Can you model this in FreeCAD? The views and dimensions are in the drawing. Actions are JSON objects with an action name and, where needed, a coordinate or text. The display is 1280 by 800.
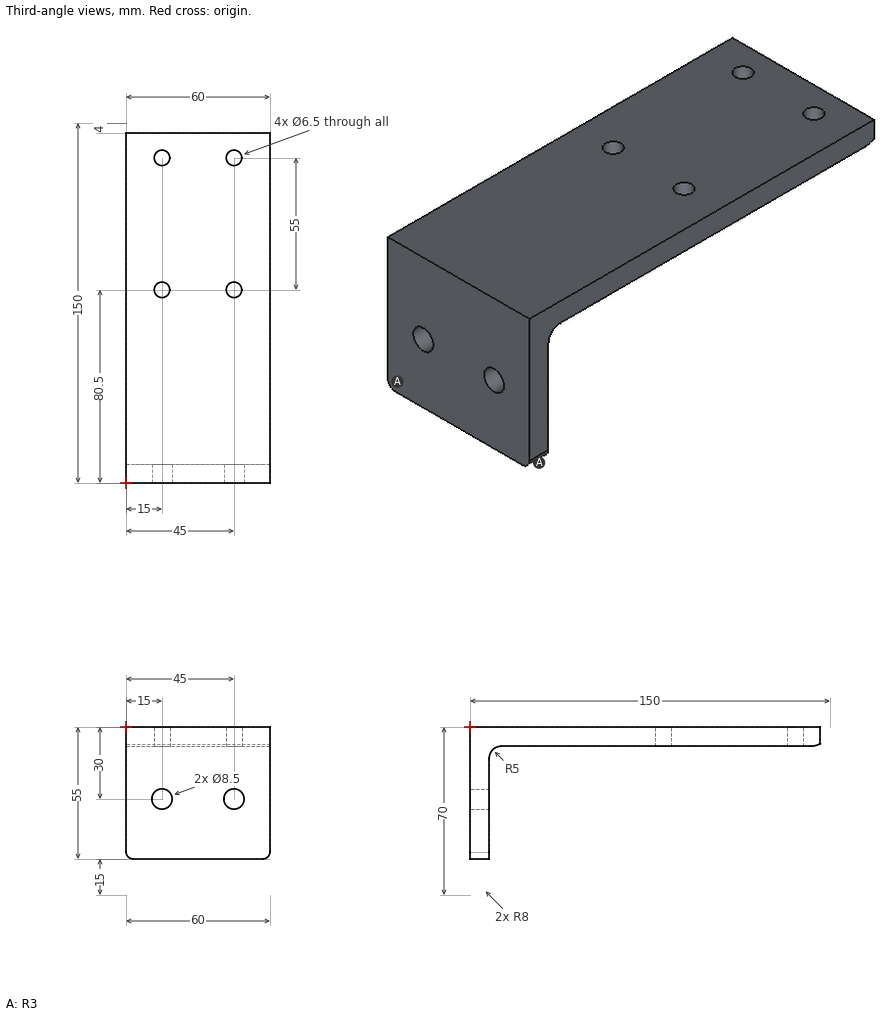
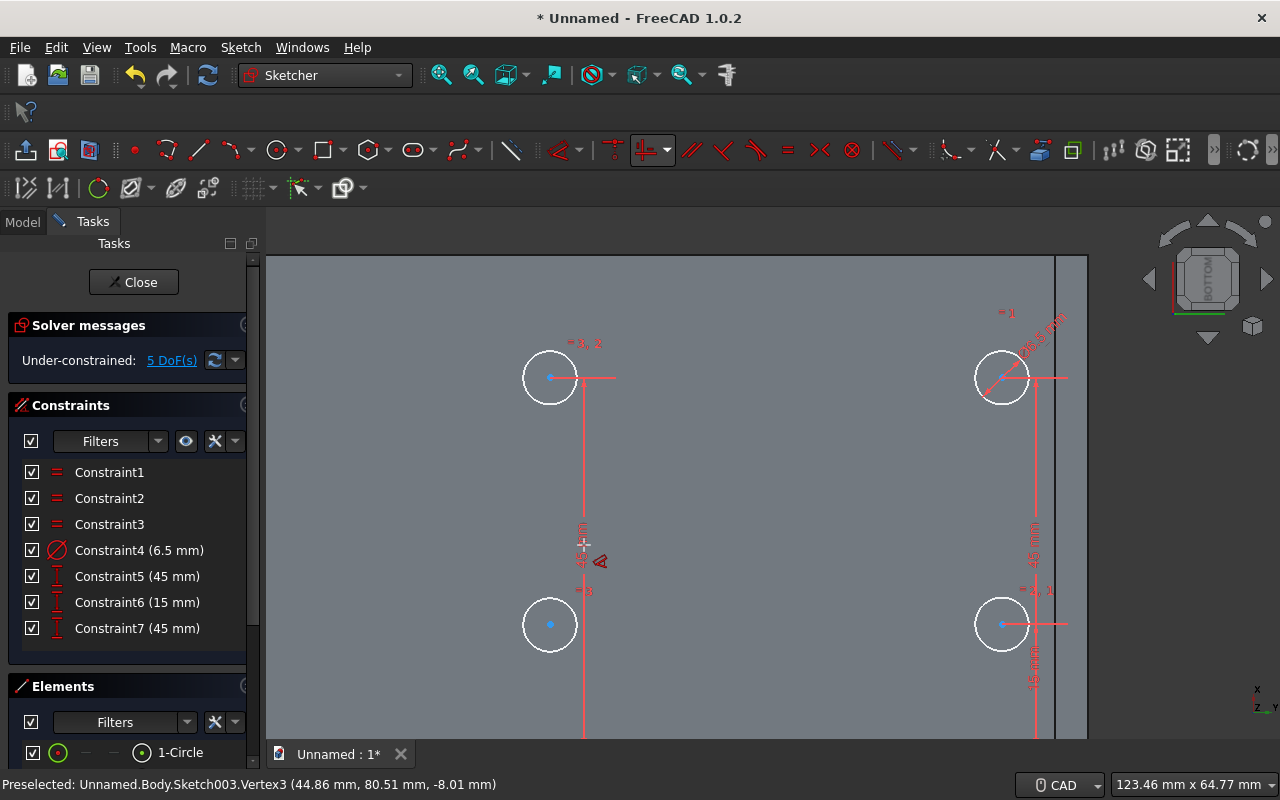
{"action": "left_click", "coordinate": [550, 625]}
{"action": "left_click", "coordinate": [584, 668]}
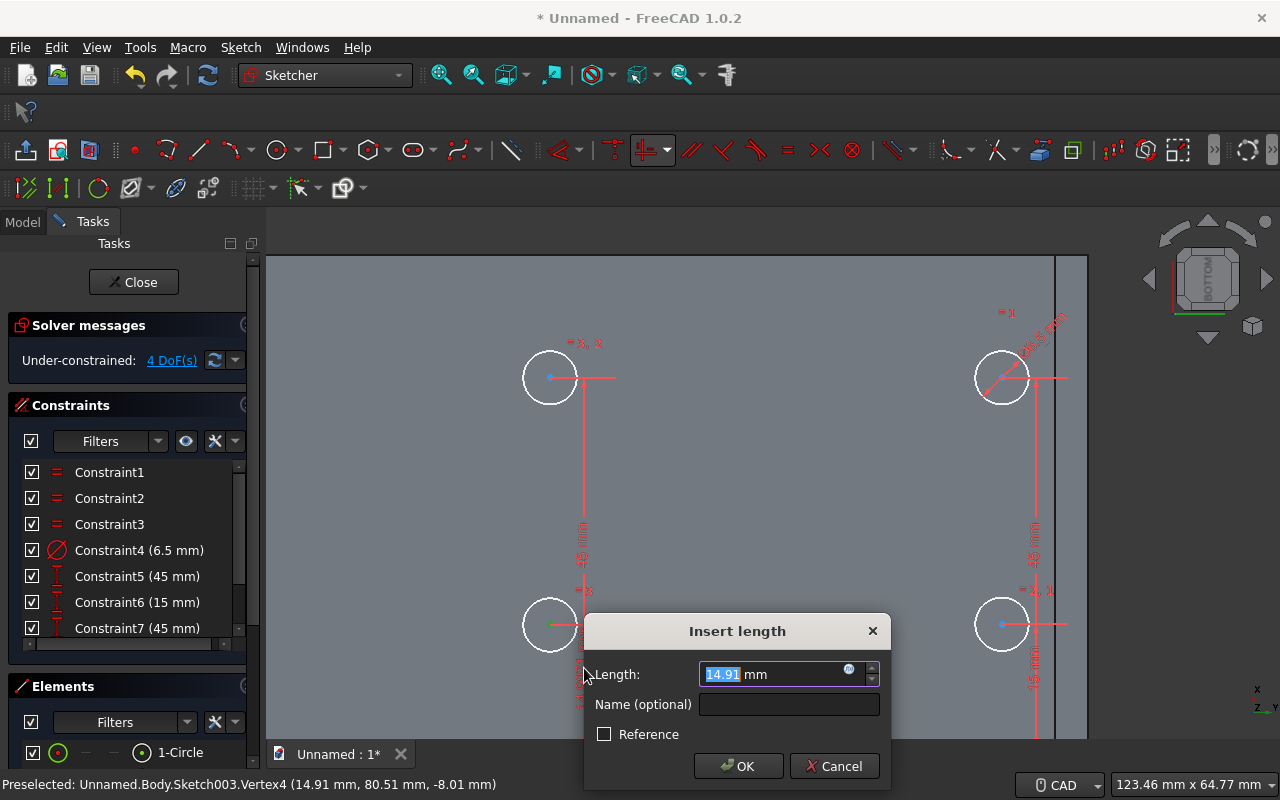
{"action": "type", "text": "15"}
{"action": "key", "text": "Return"}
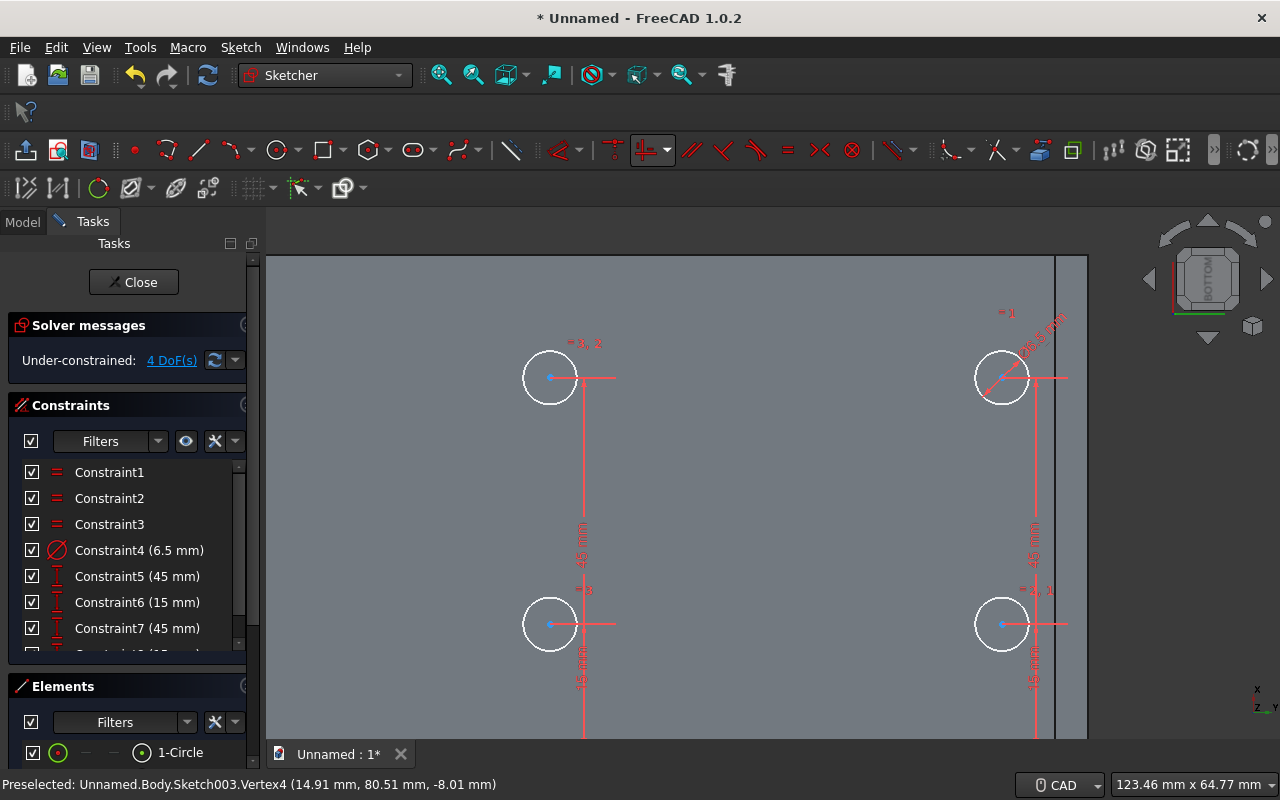
{"action": "left_click", "coordinate": [1002, 378]}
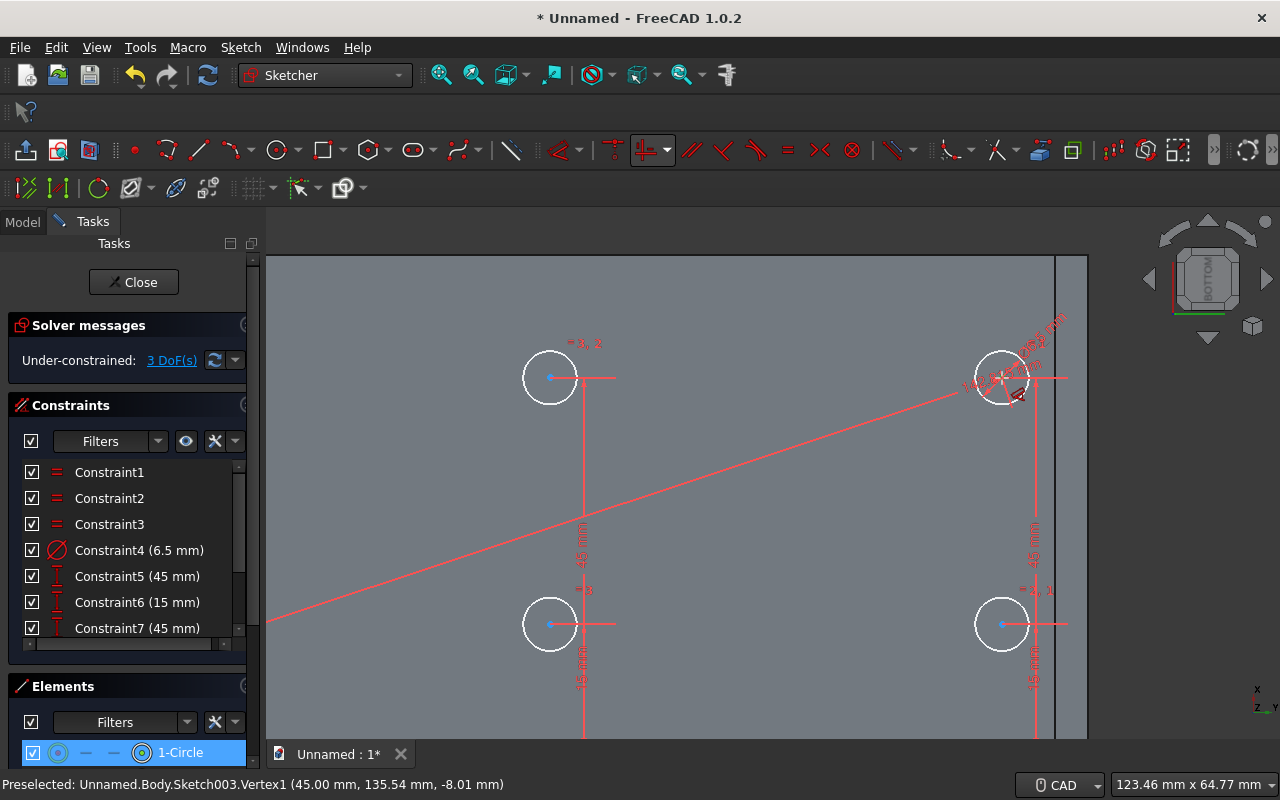
{"action": "left_click", "coordinate": [550, 378]}
{"action": "left_click", "coordinate": [776, 344]}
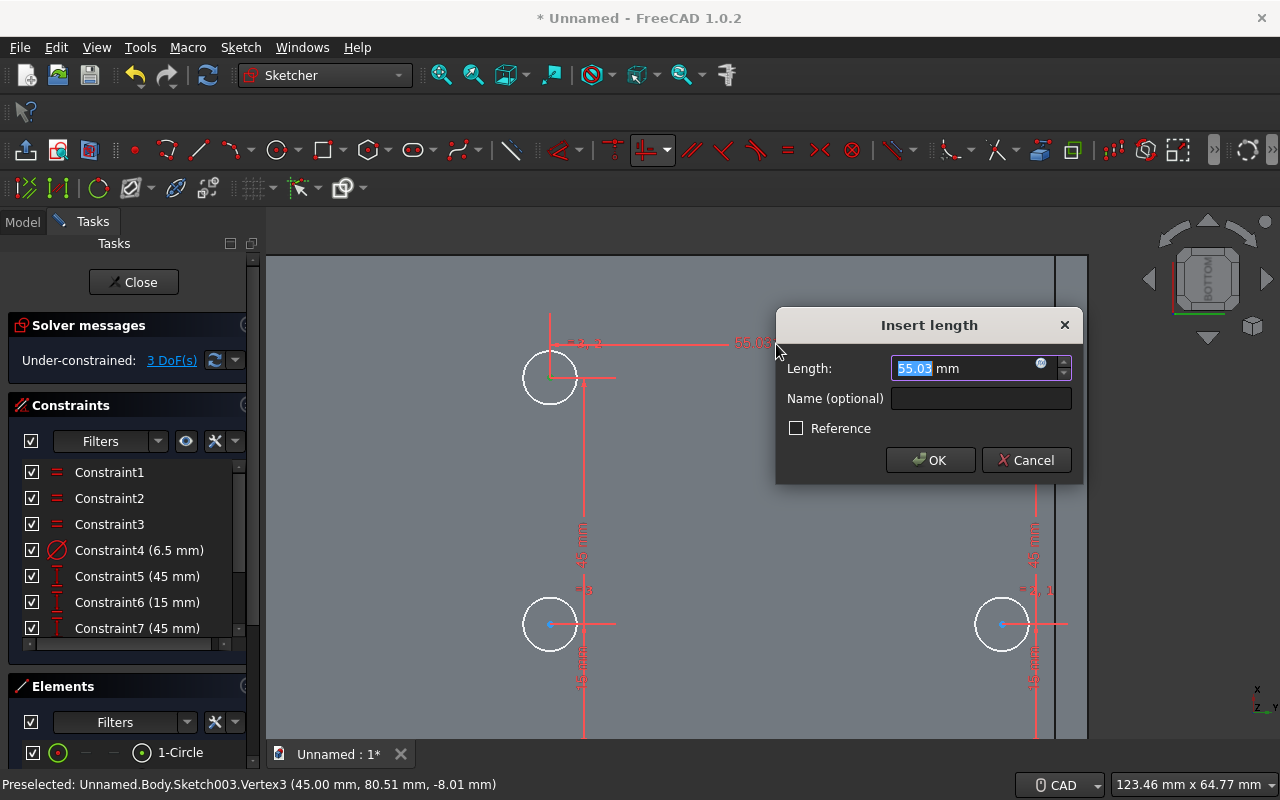
{"action": "type", "text": "55"}
{"action": "key", "text": "Return"}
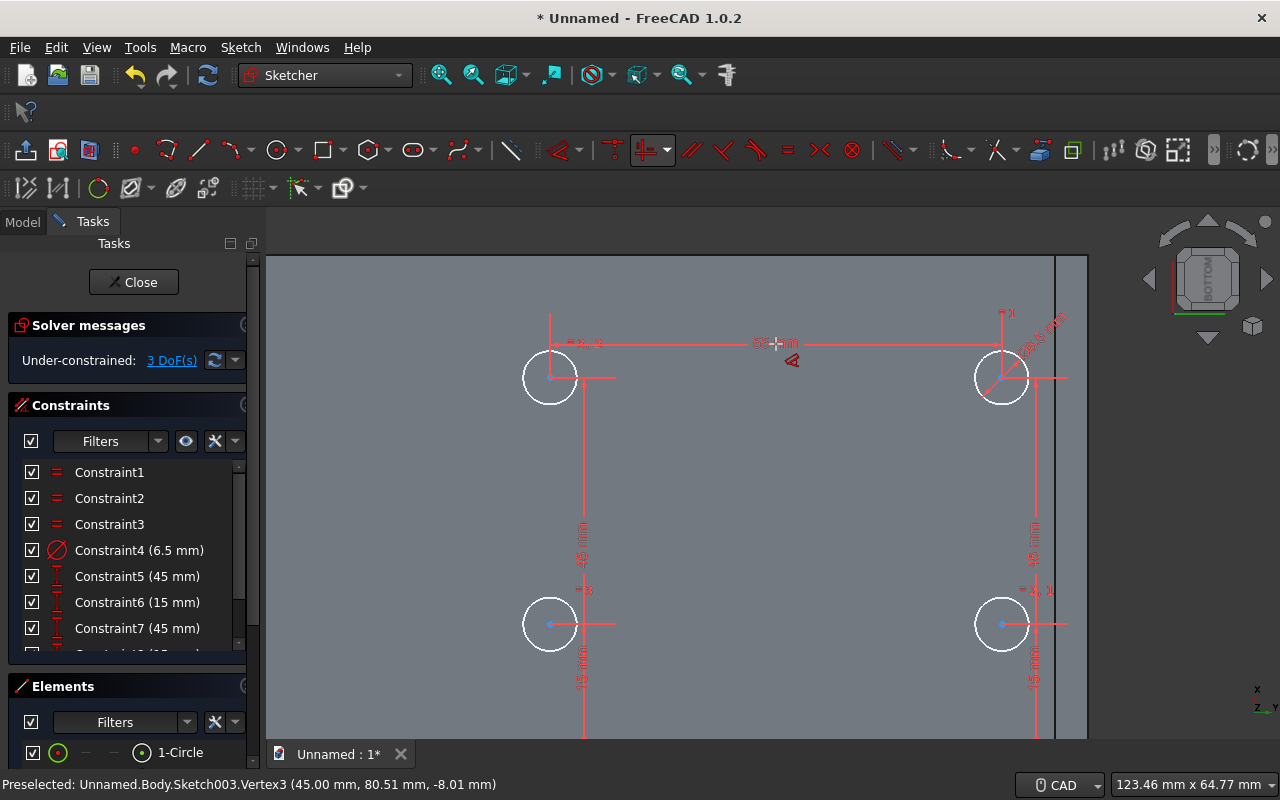
{"action": "left_click", "coordinate": [1002, 624]}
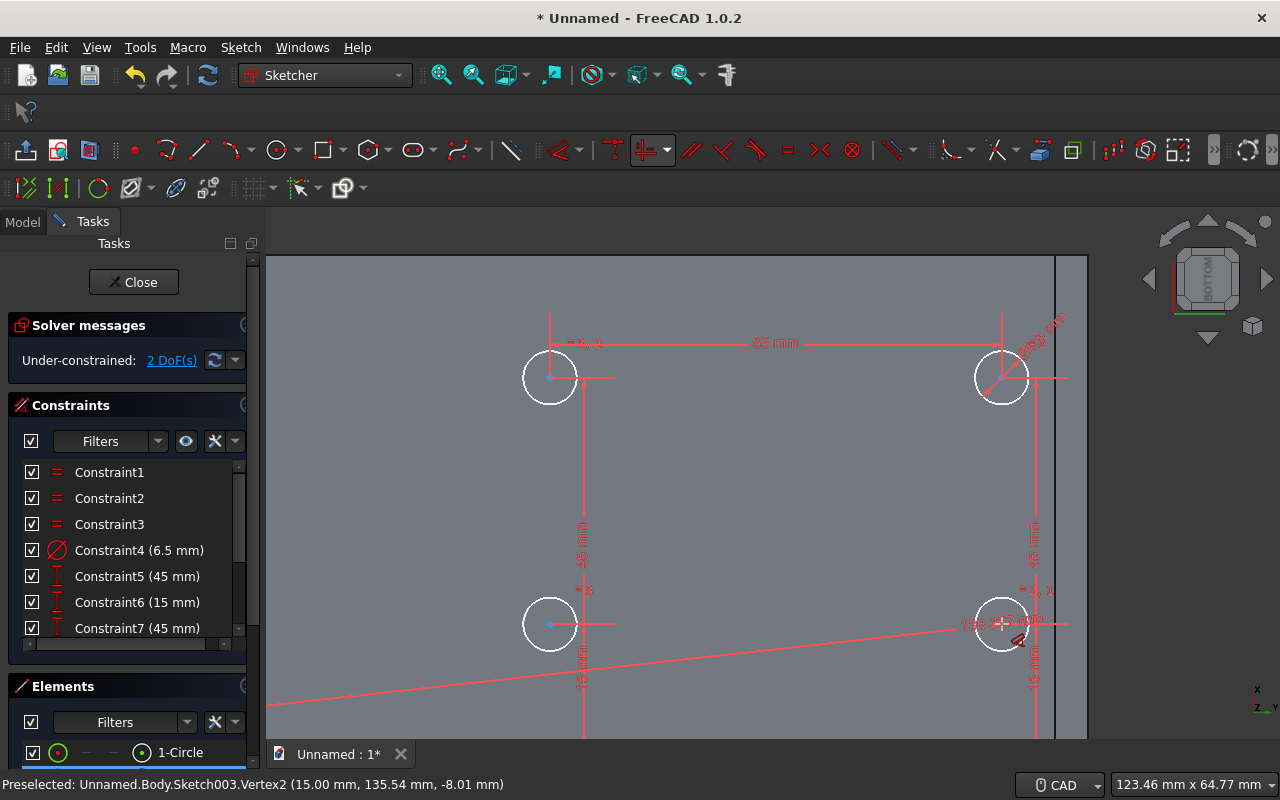
{"action": "left_click", "coordinate": [550, 378]}
{"action": "left_click", "coordinate": [672, 344]}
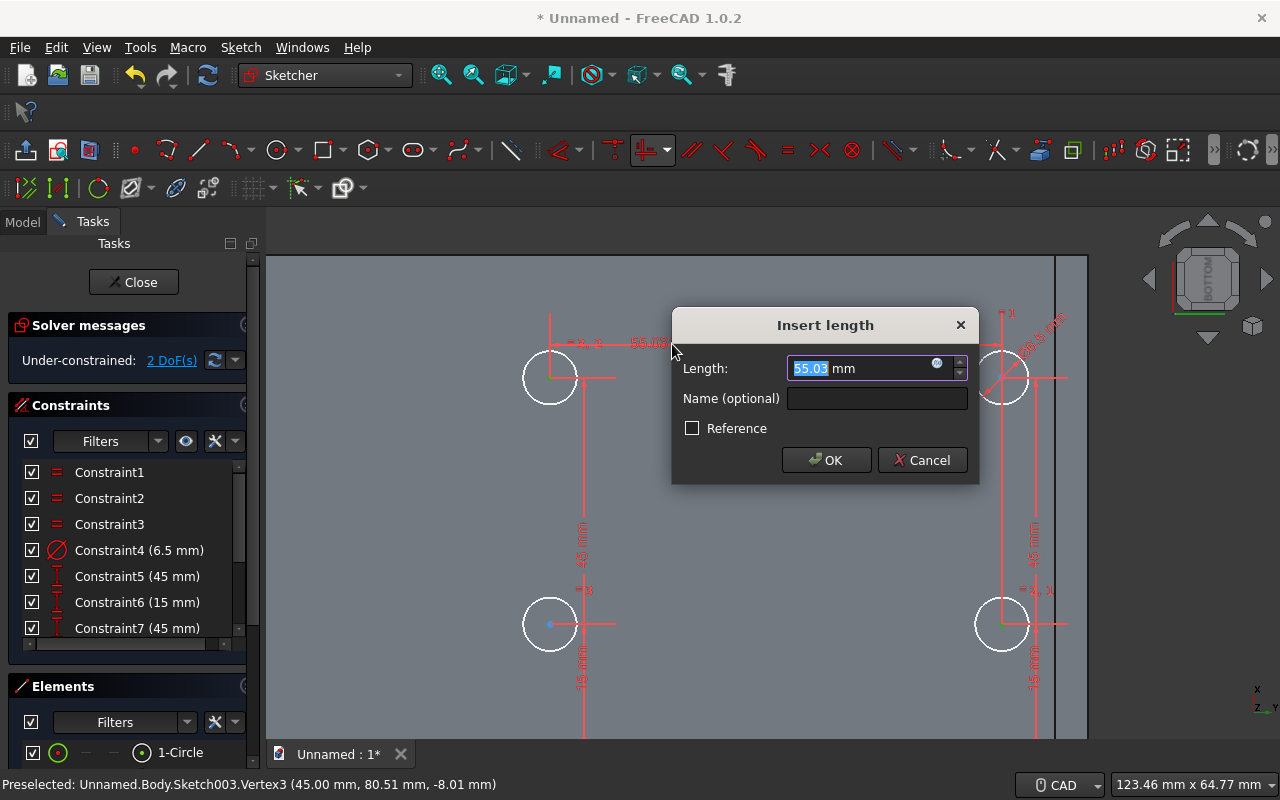
{"action": "type", "text": "55"}
{"action": "key", "text": "Return"}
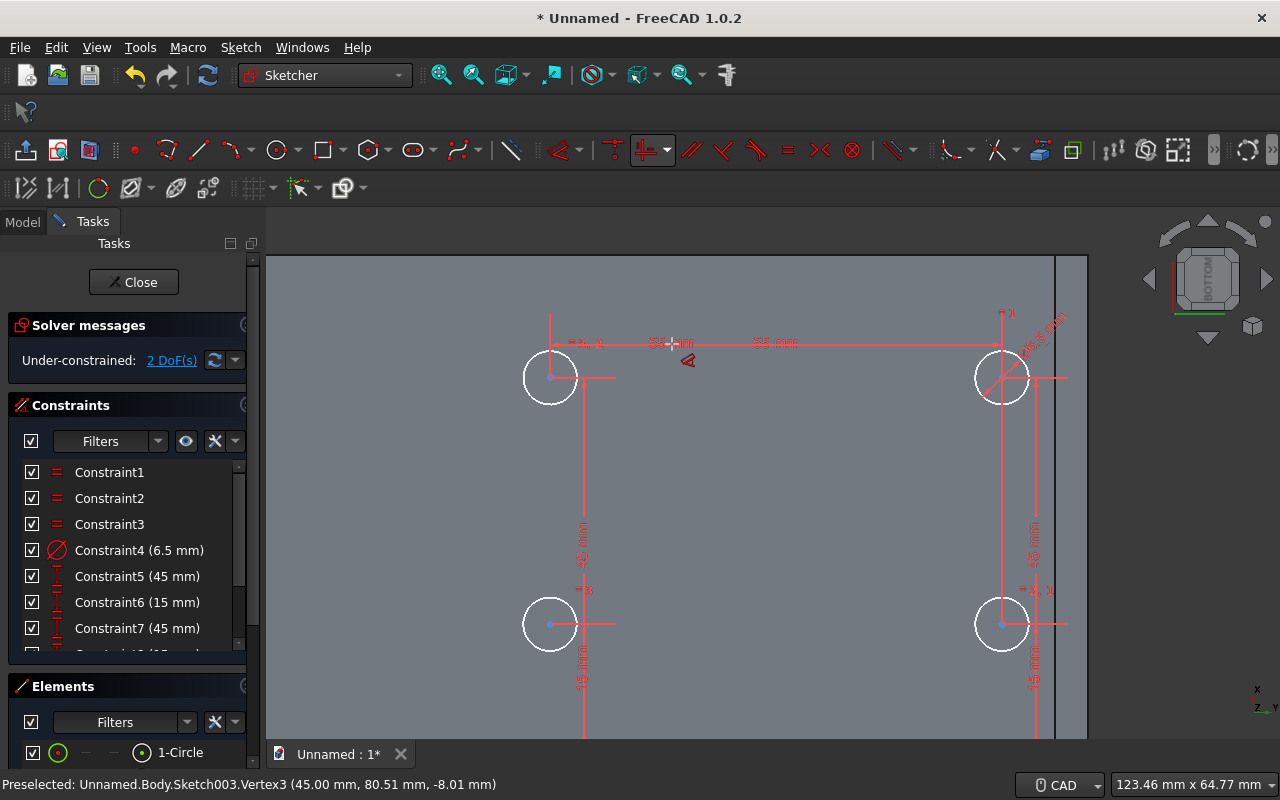
{"action": "left_click", "coordinate": [1002, 624]}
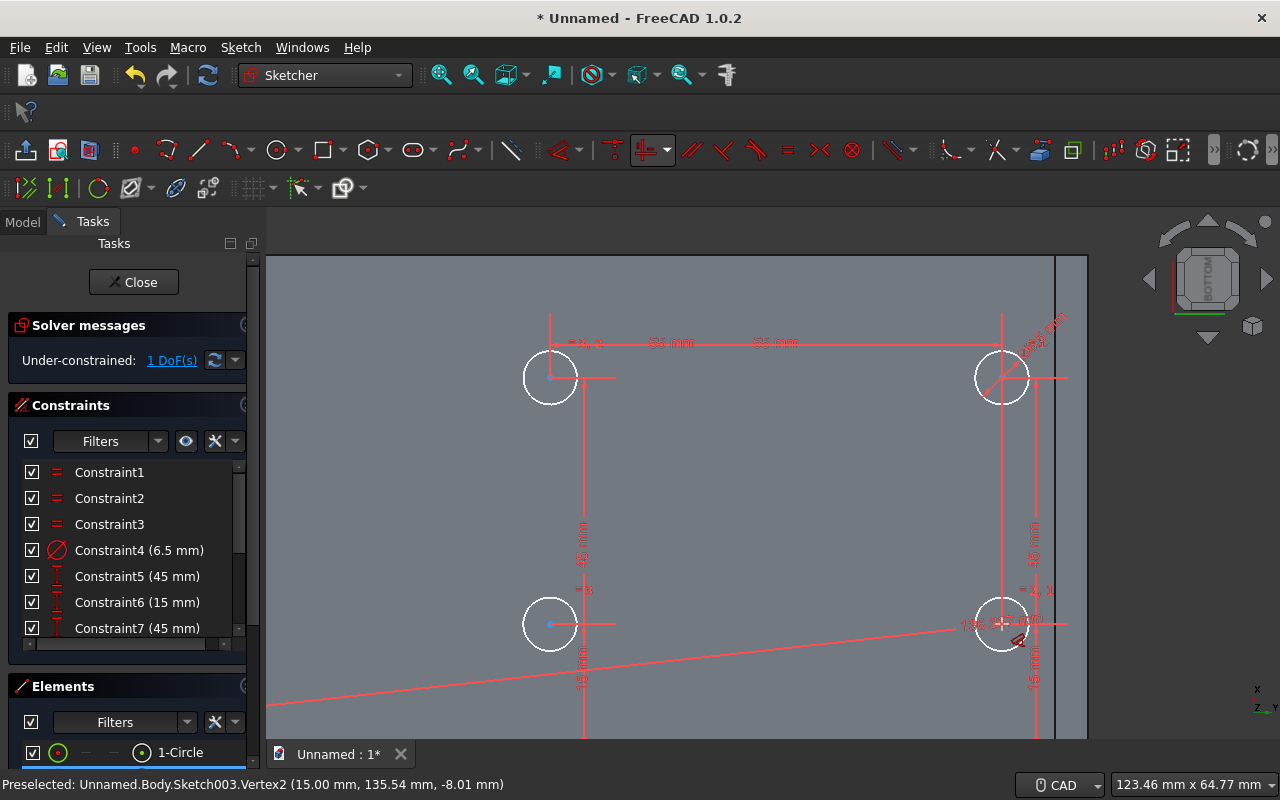
{"action": "left_click", "coordinate": [550, 624]}
{"action": "left_click", "coordinate": [776, 658]}